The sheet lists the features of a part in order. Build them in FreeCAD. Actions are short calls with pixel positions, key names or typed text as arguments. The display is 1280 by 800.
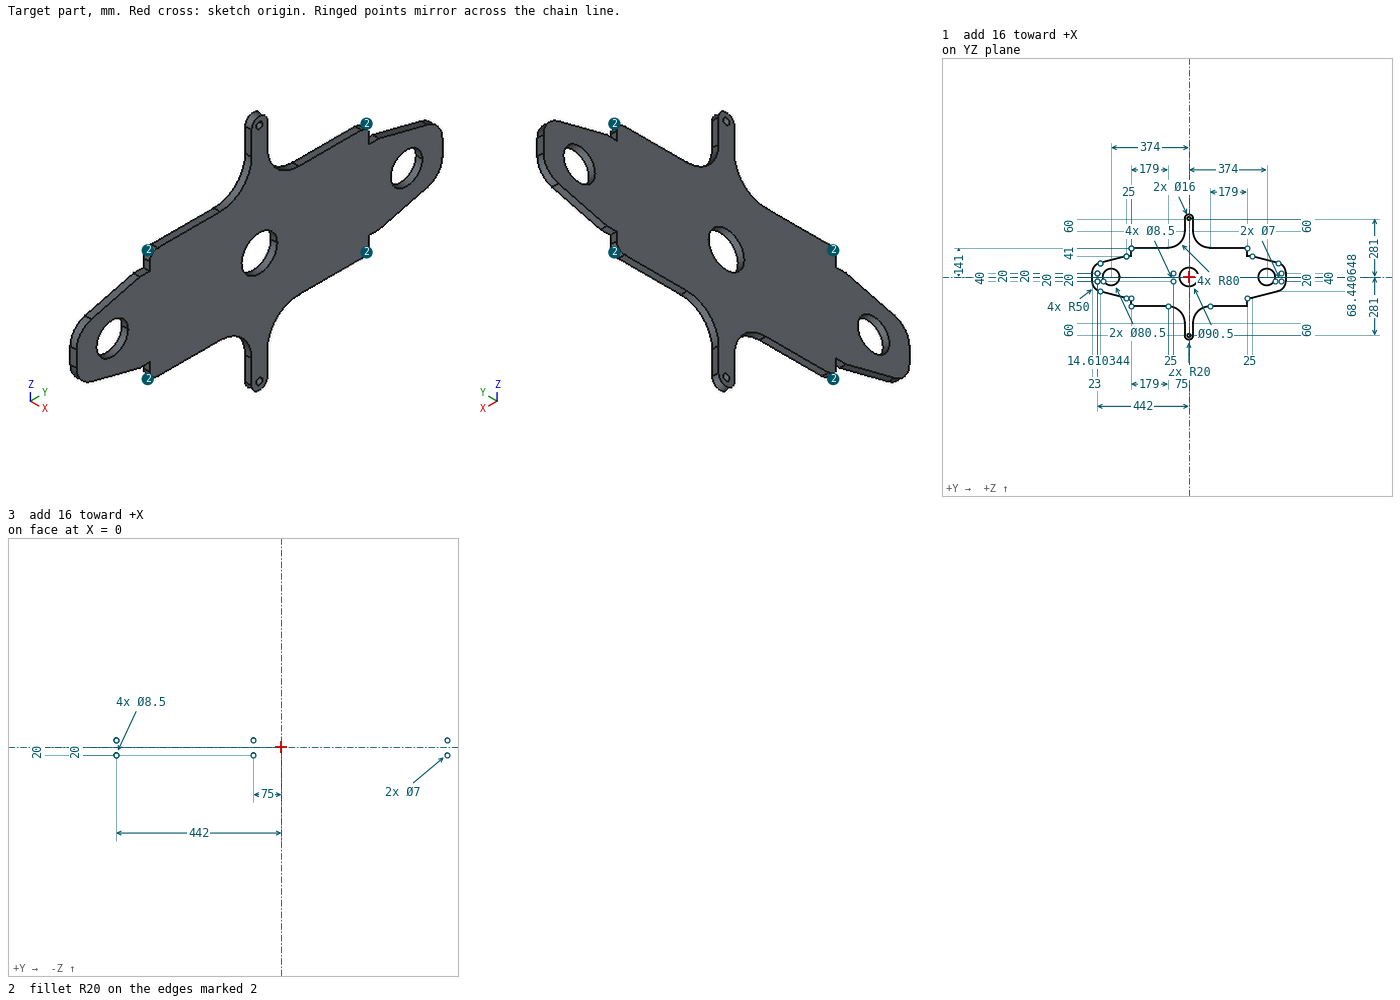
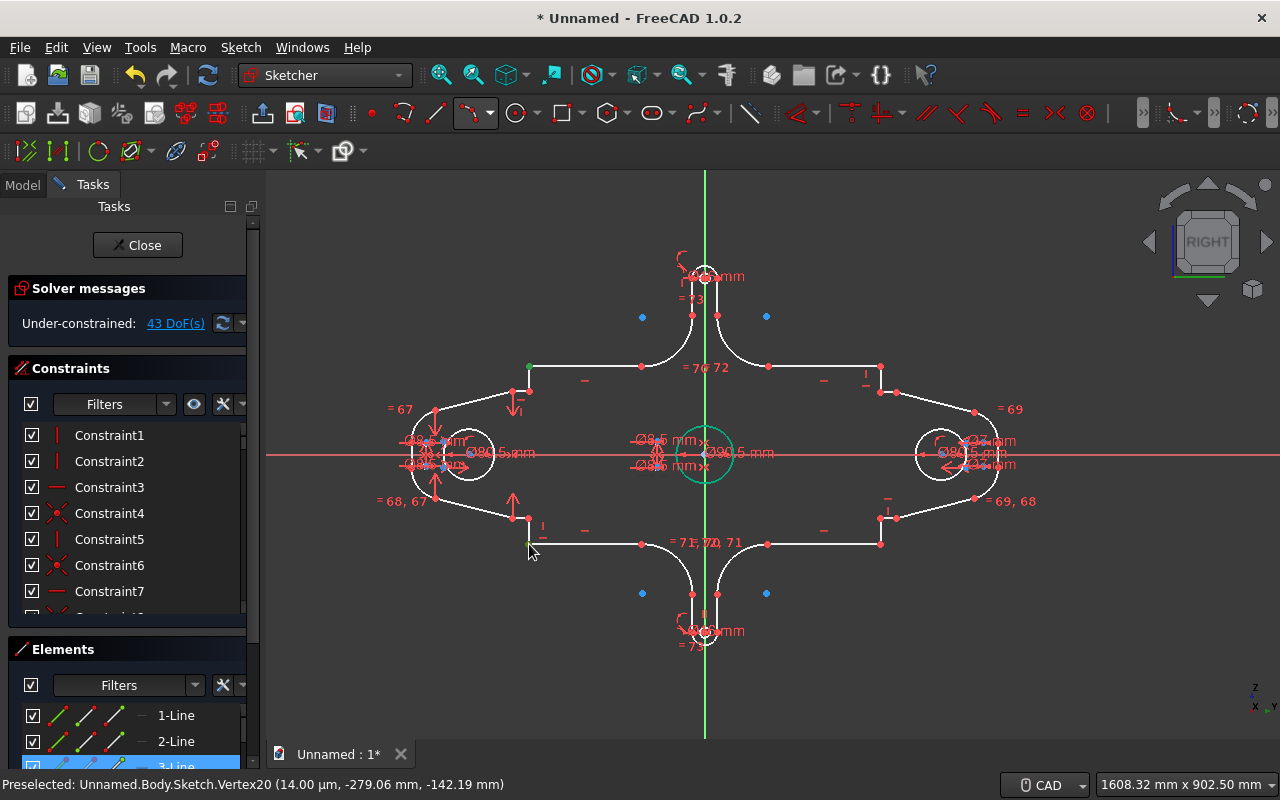
click(353, 455)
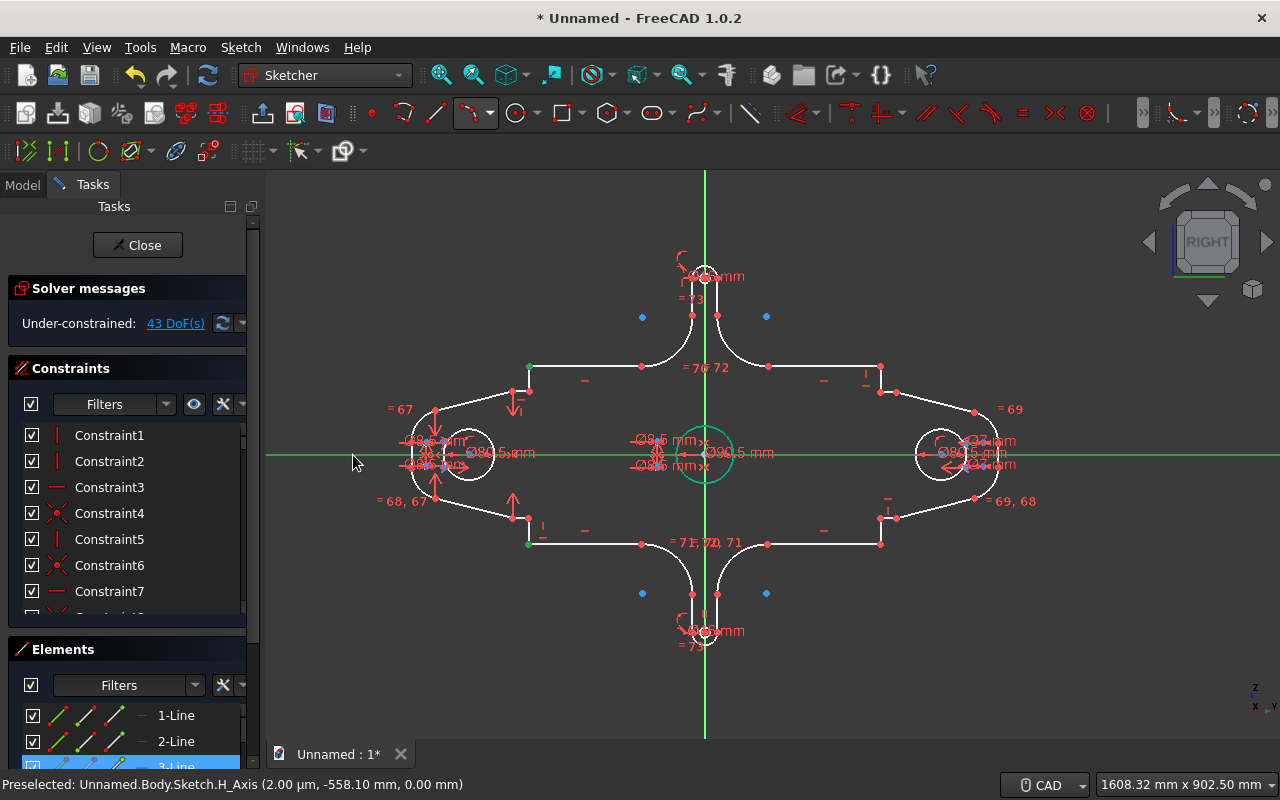
key(s)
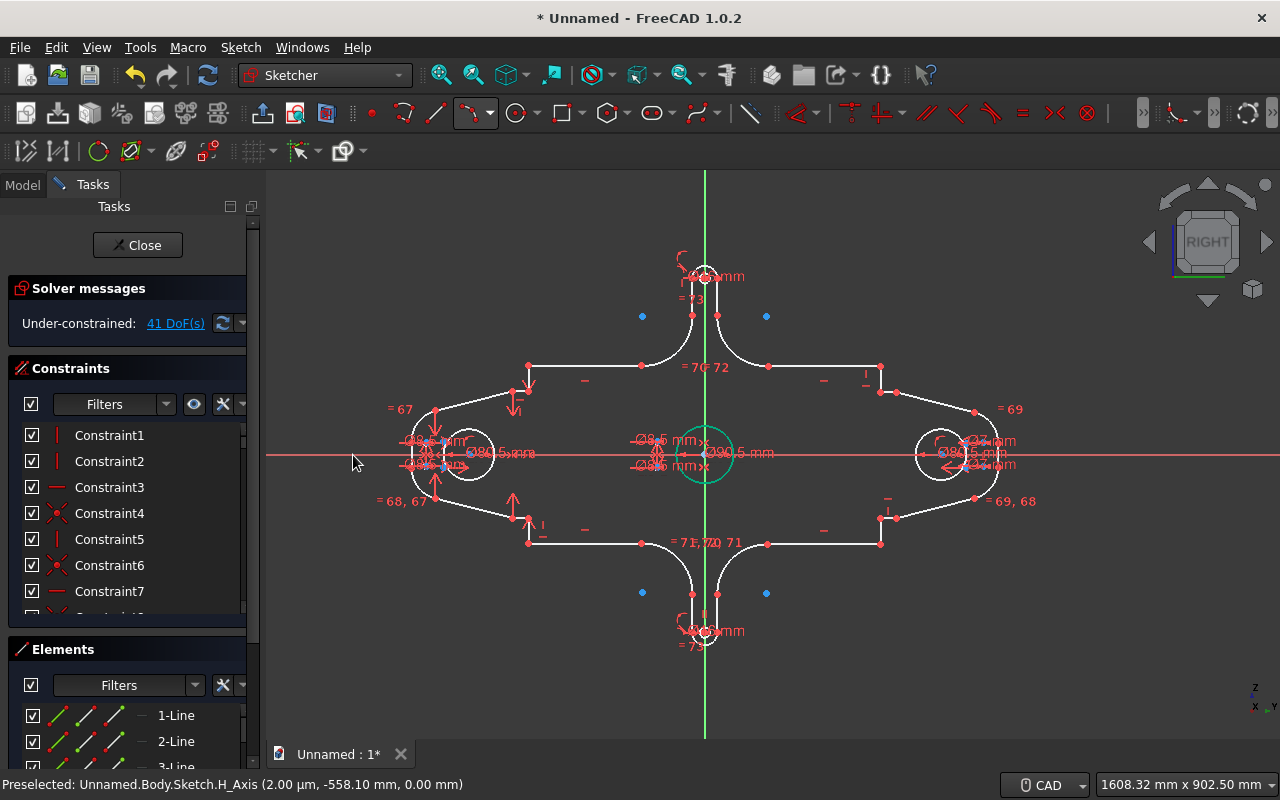
click(642, 544)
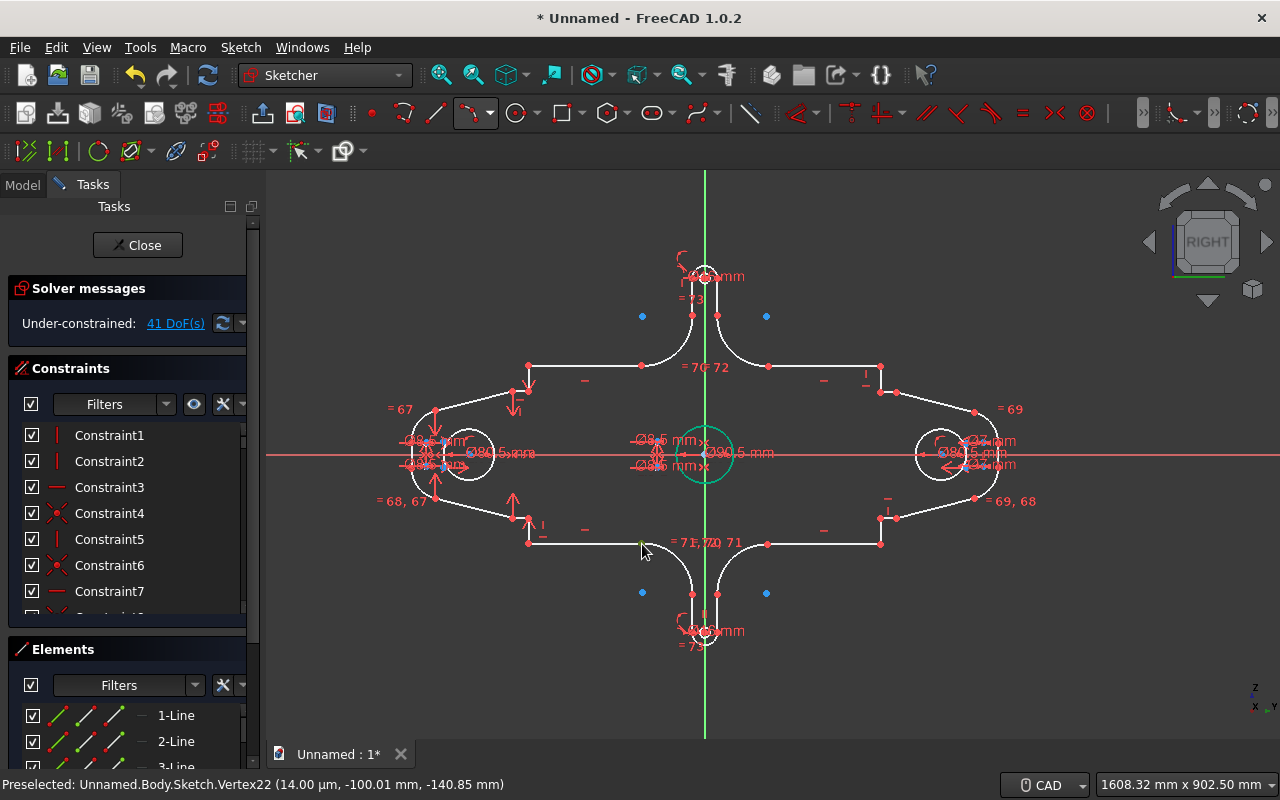
click(768, 544)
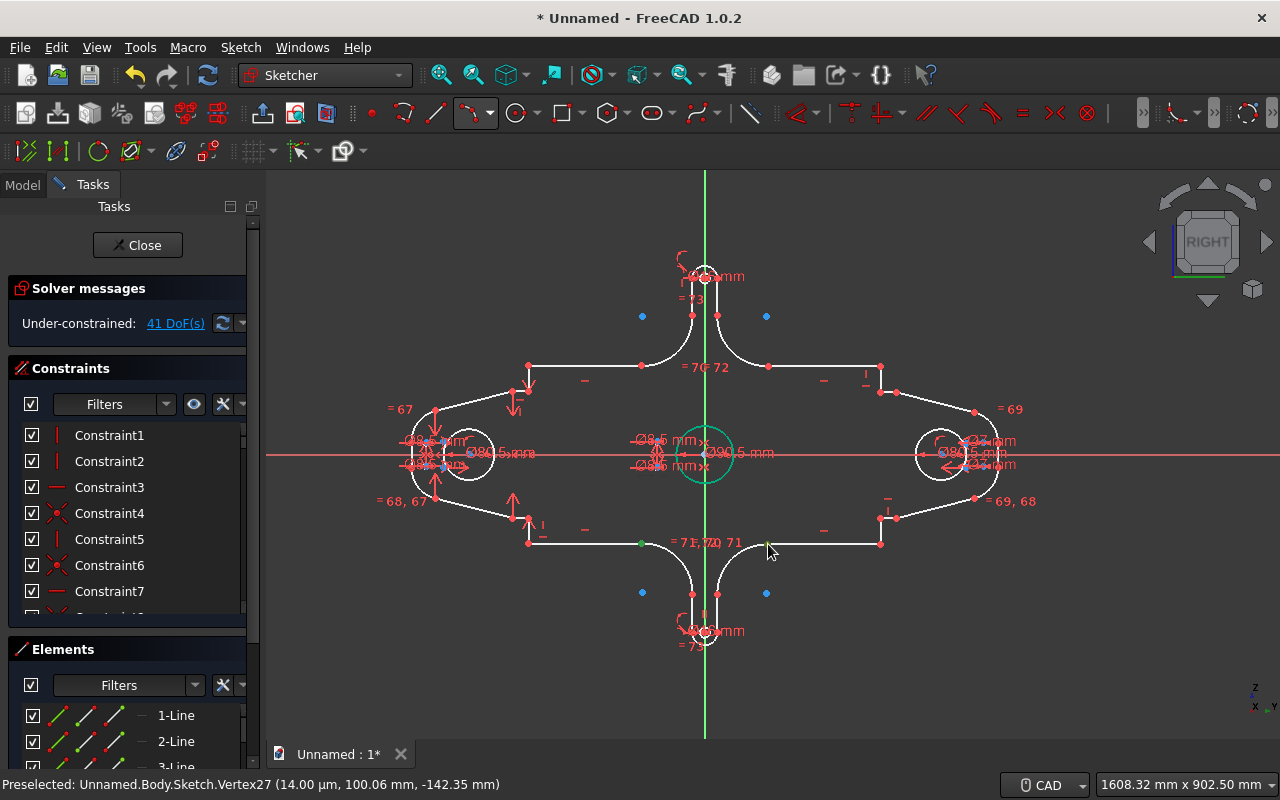
click(705, 528)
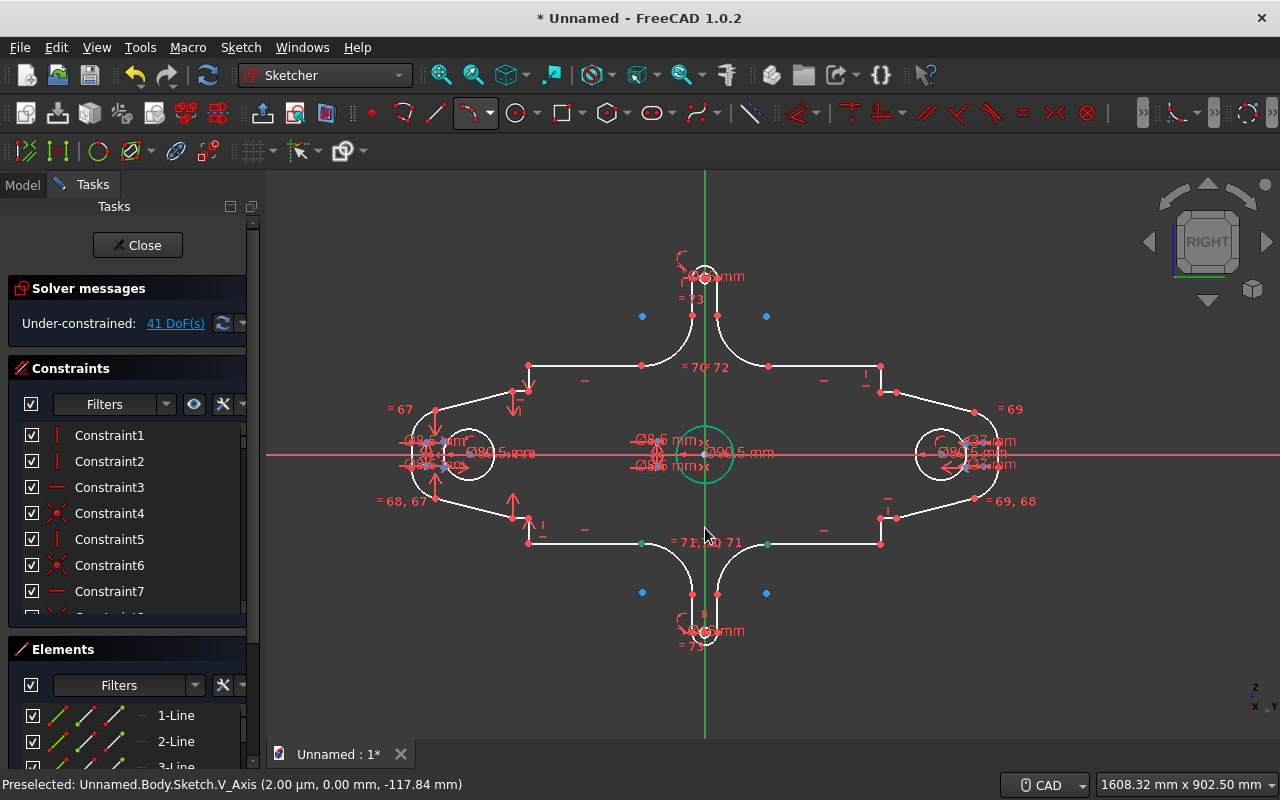
click(1056, 114)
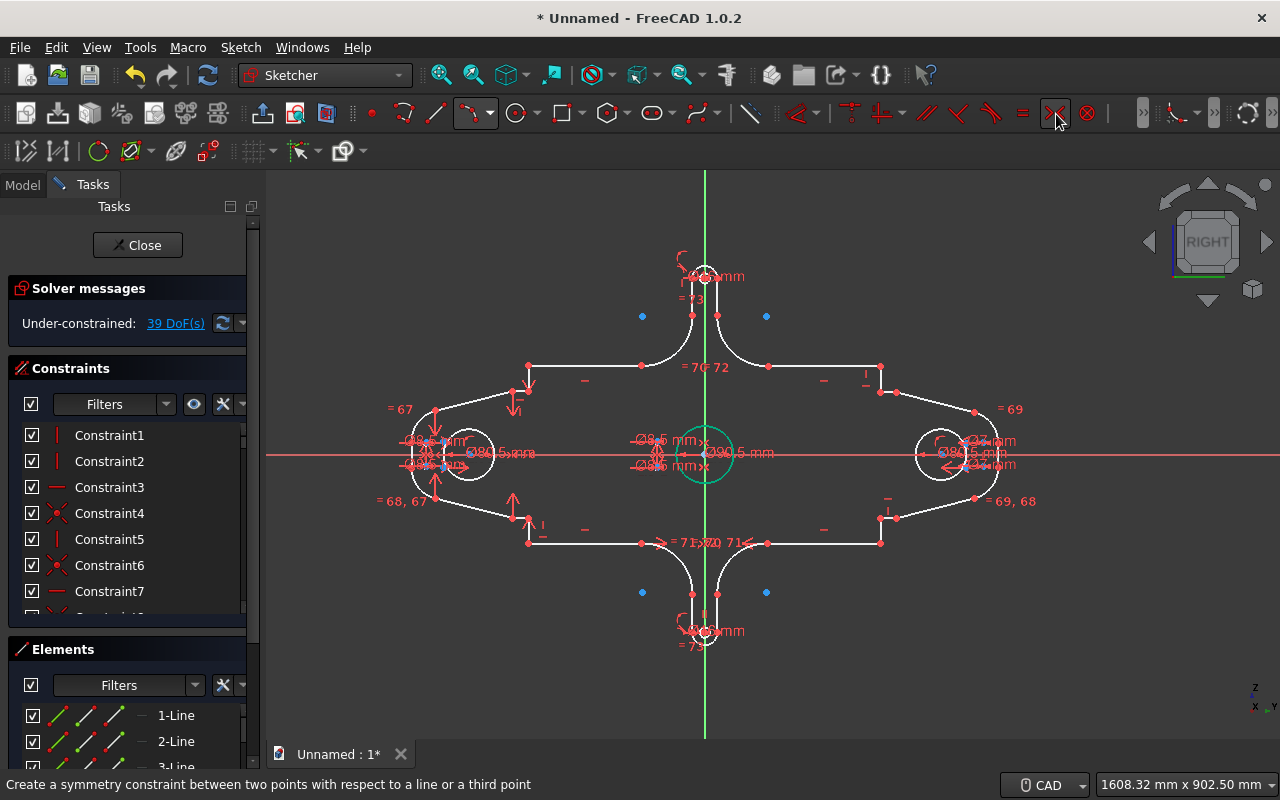
click(529, 518)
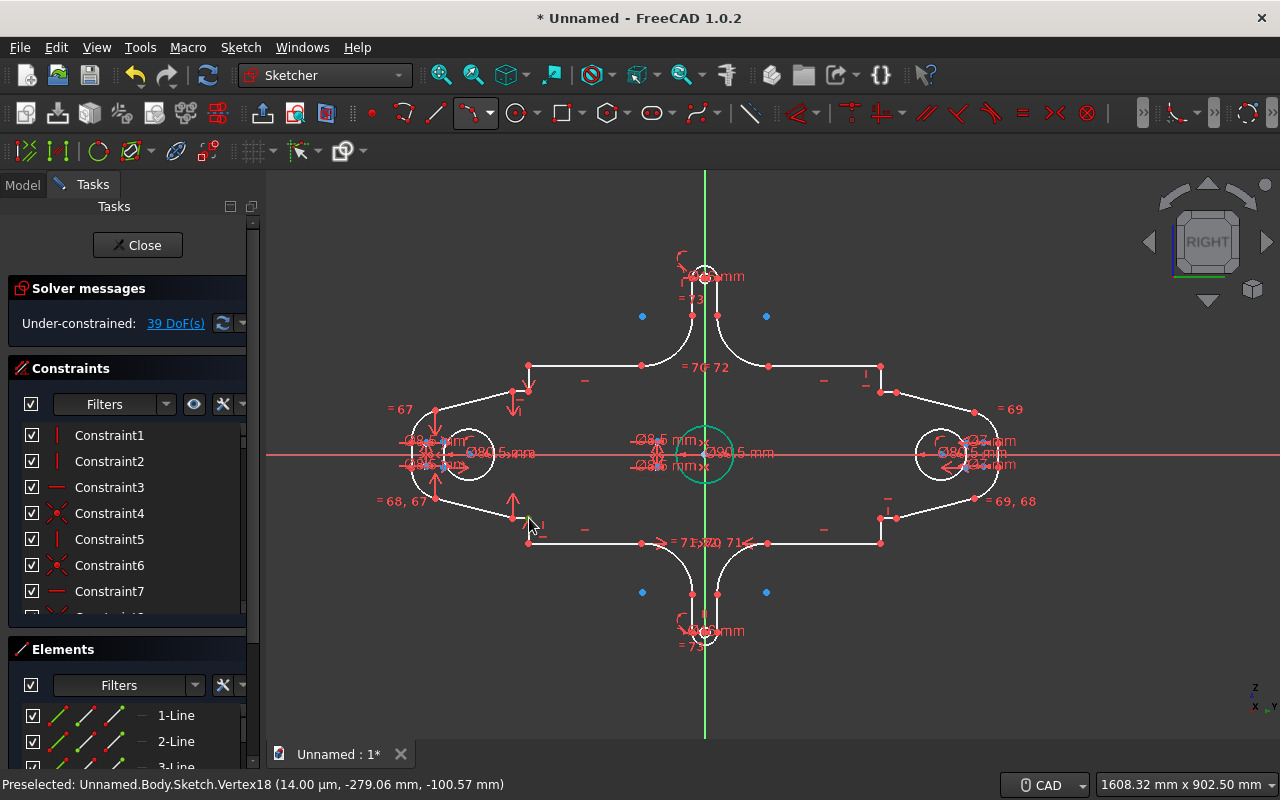
click(881, 518)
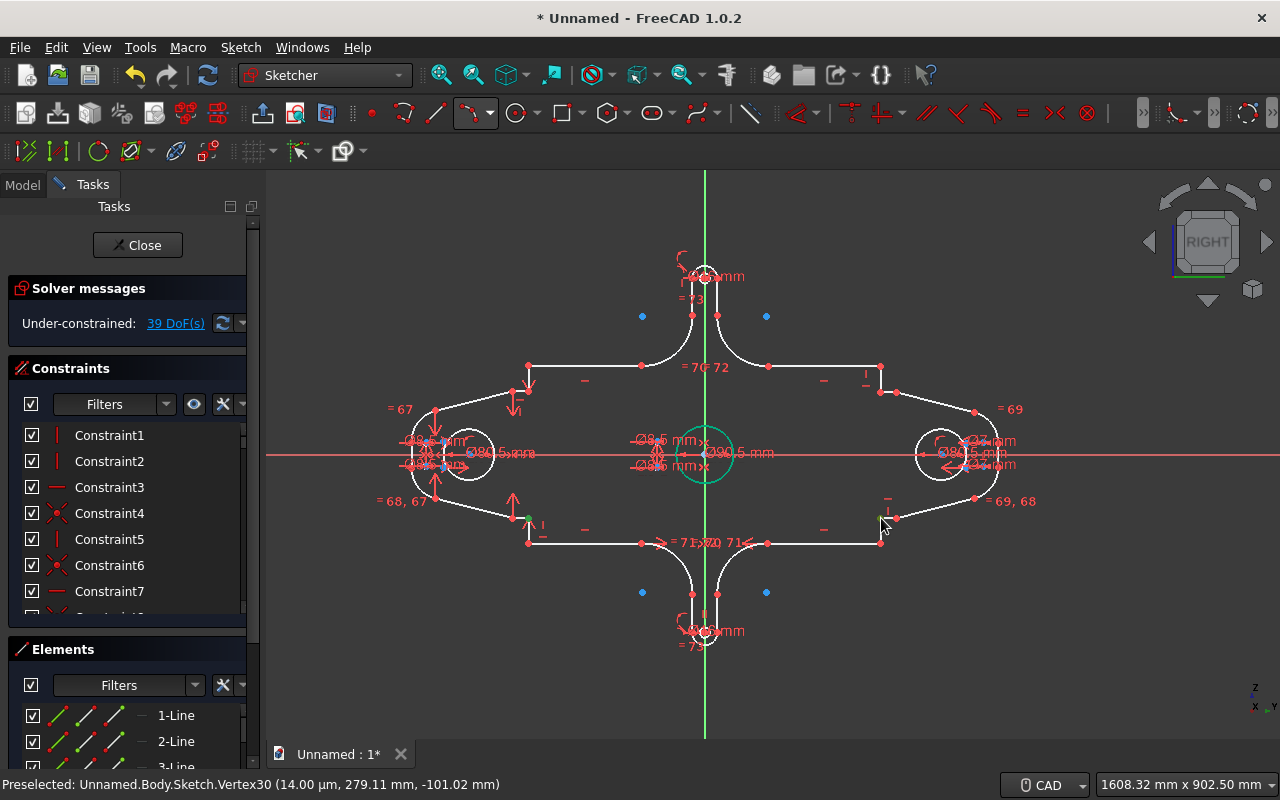
click(705, 528)